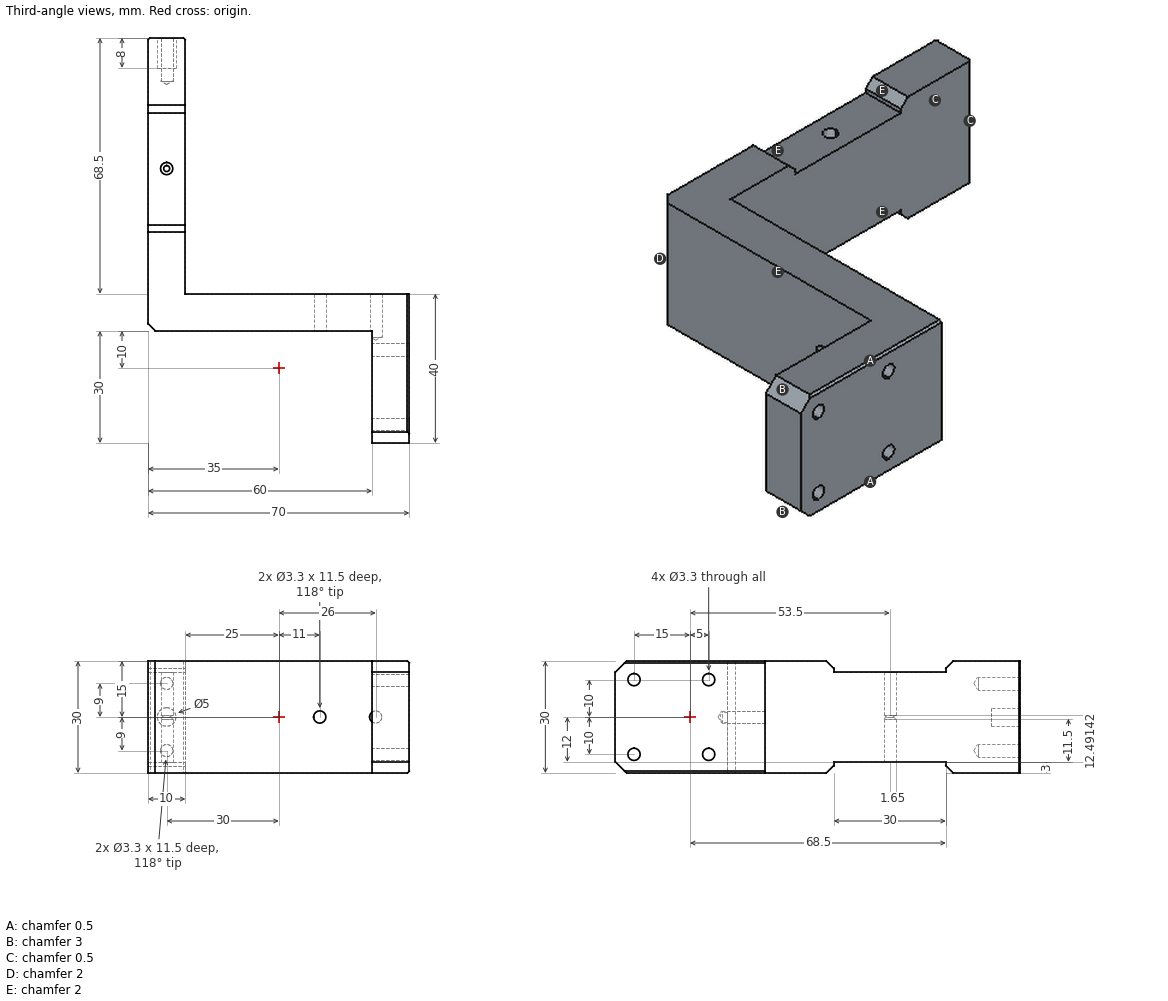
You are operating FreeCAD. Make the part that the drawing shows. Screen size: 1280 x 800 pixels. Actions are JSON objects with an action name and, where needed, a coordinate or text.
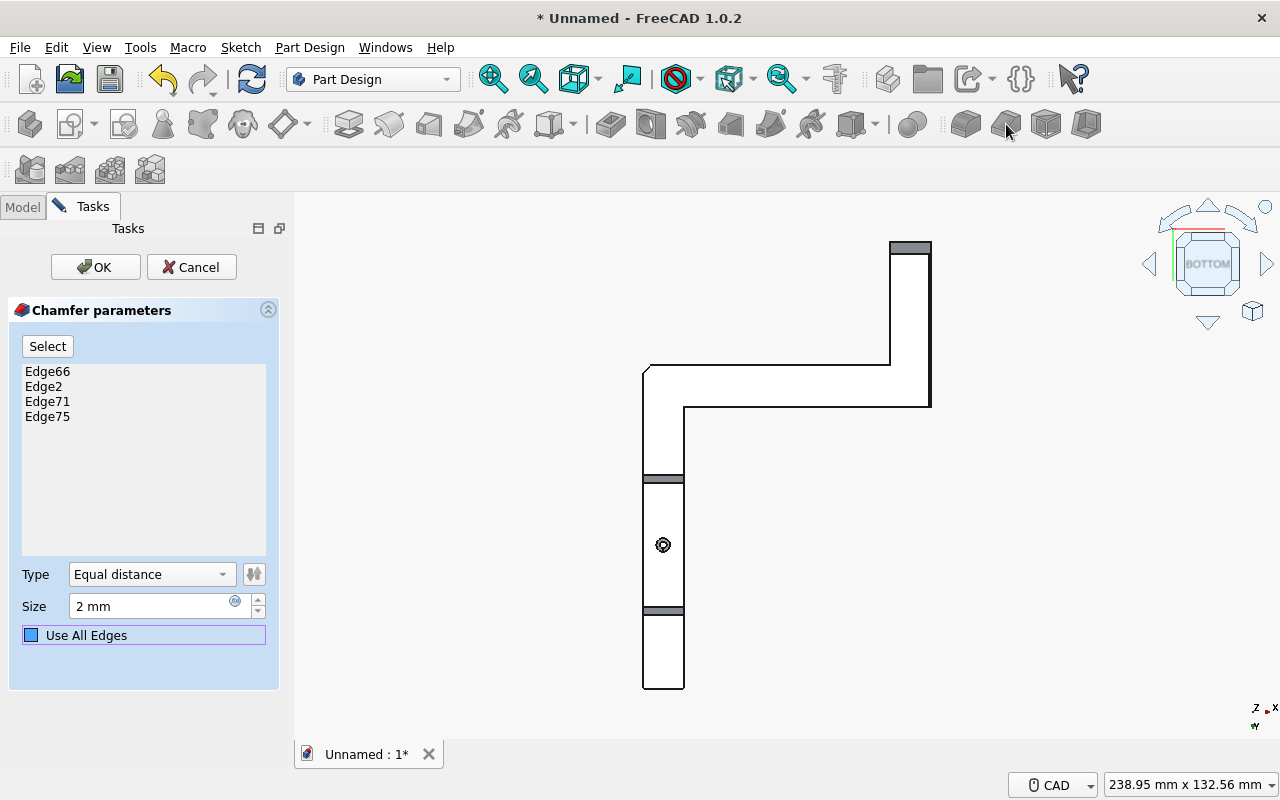
{"action": "left_click", "coordinate": [96, 267]}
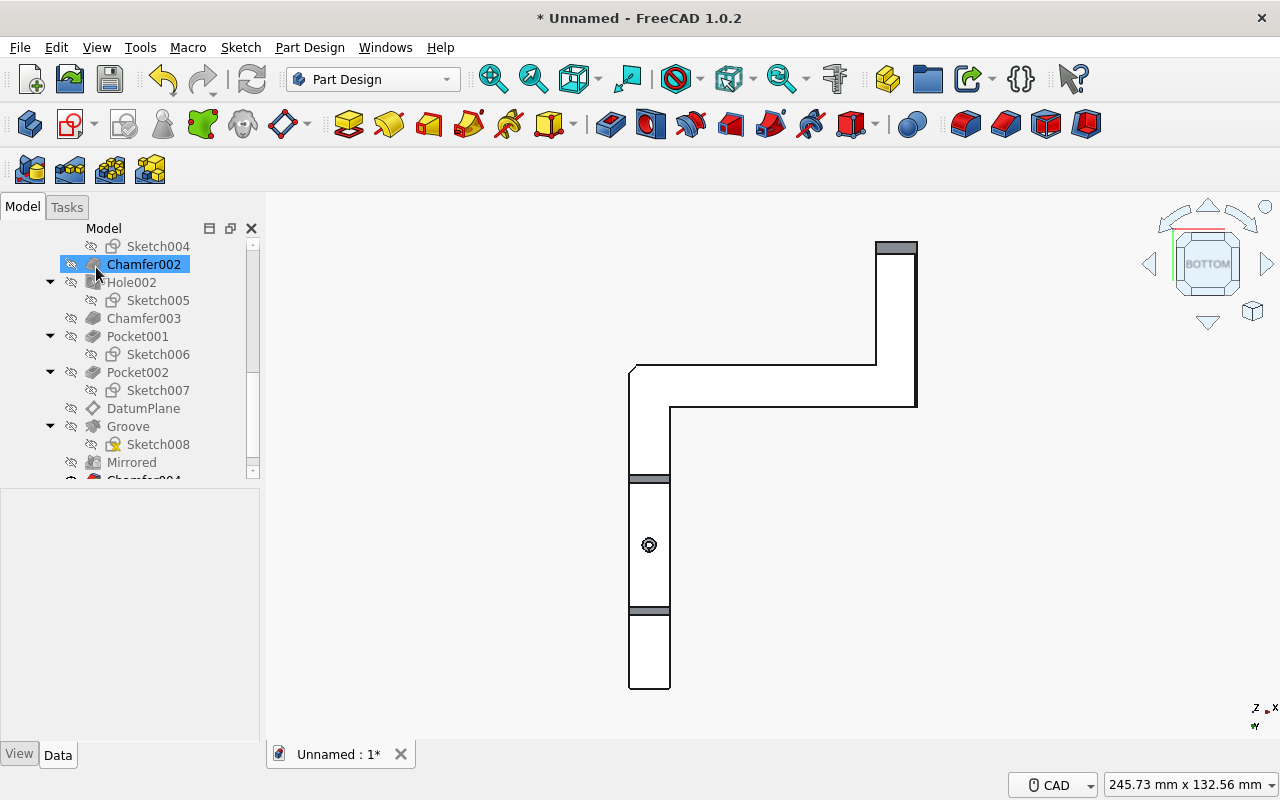
{"action": "key", "text": "0"}